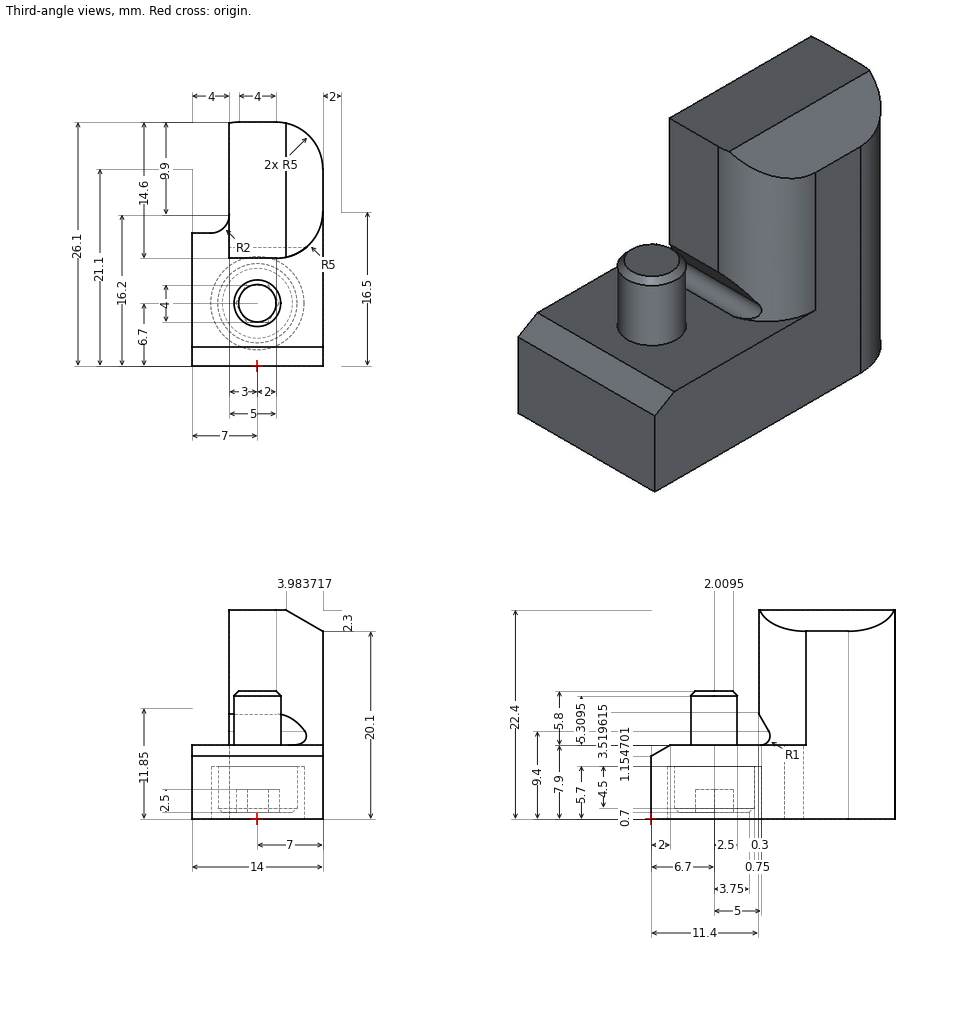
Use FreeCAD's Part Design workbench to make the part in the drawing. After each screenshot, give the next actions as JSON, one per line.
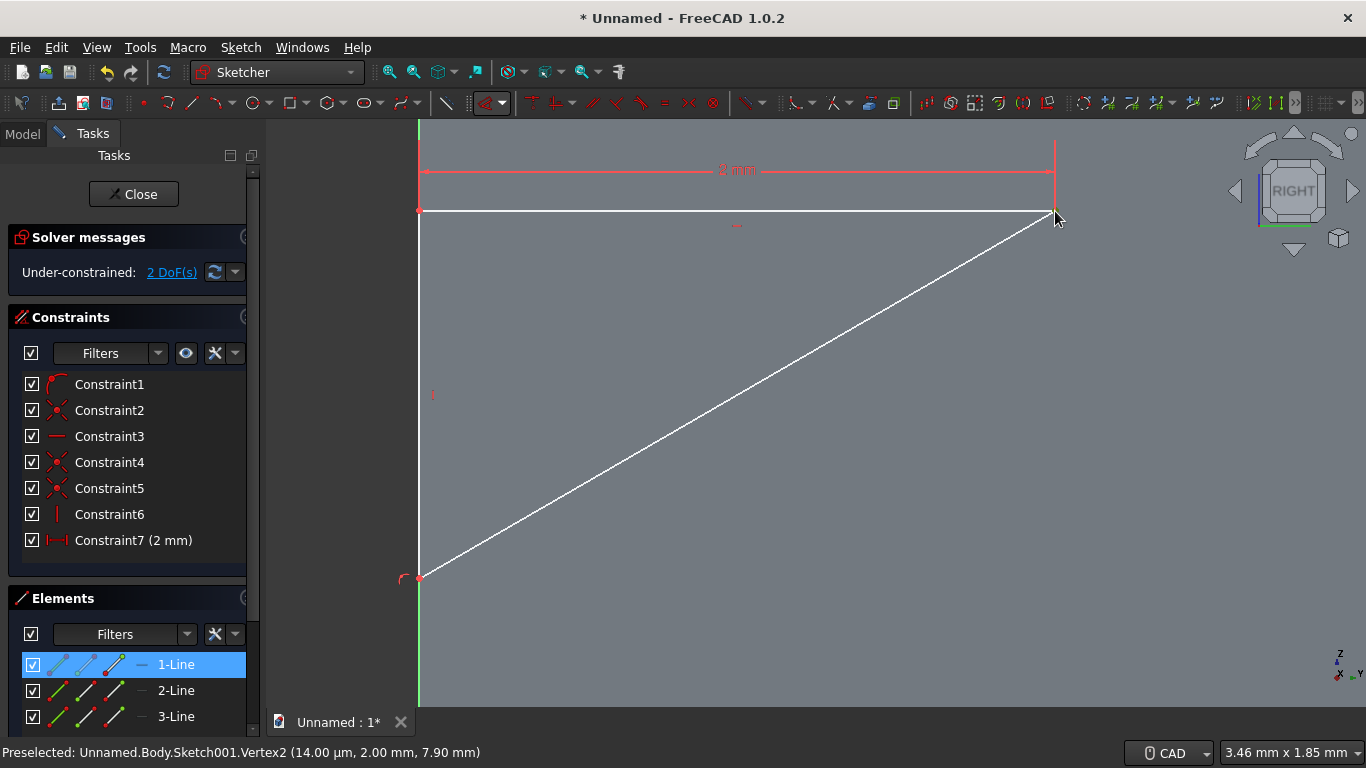
{"action": "left_click", "coordinate": [504, 104]}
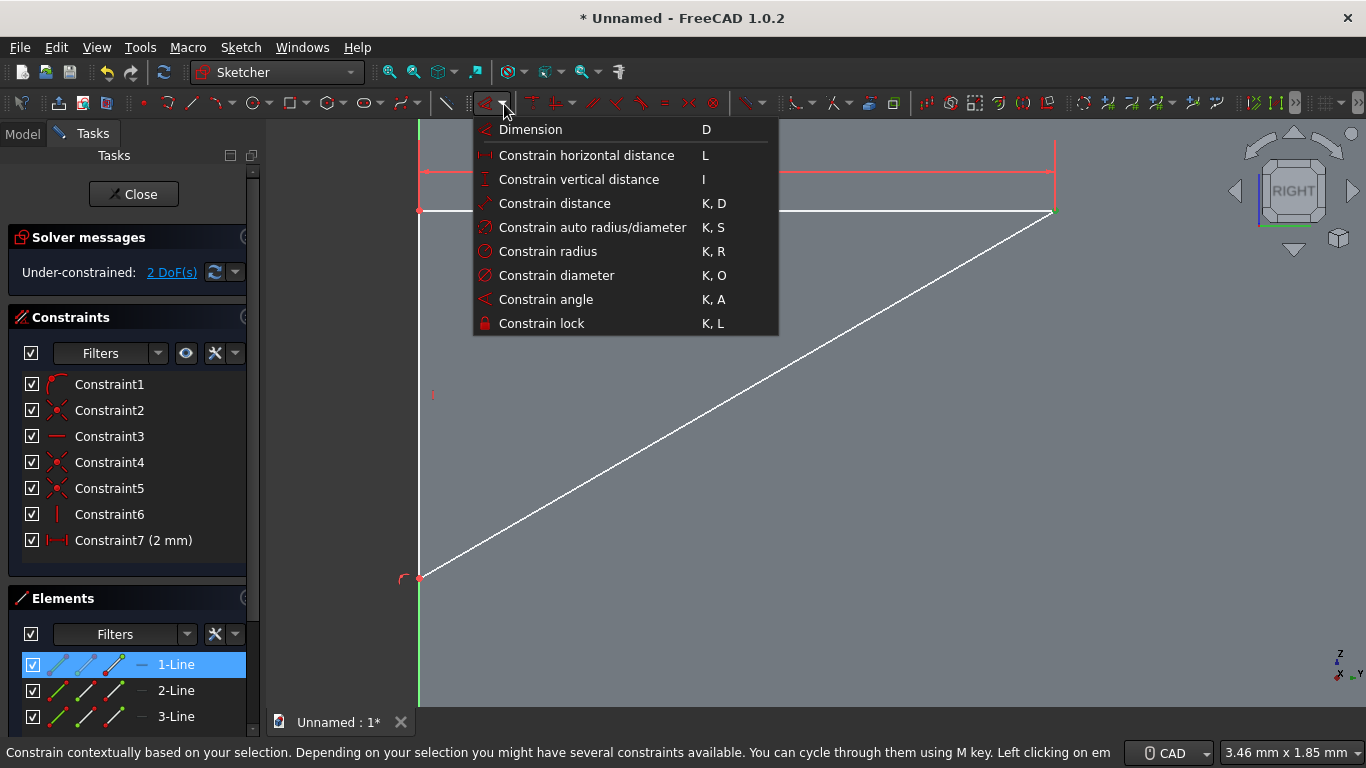
{"action": "left_click", "coordinate": [626, 179]}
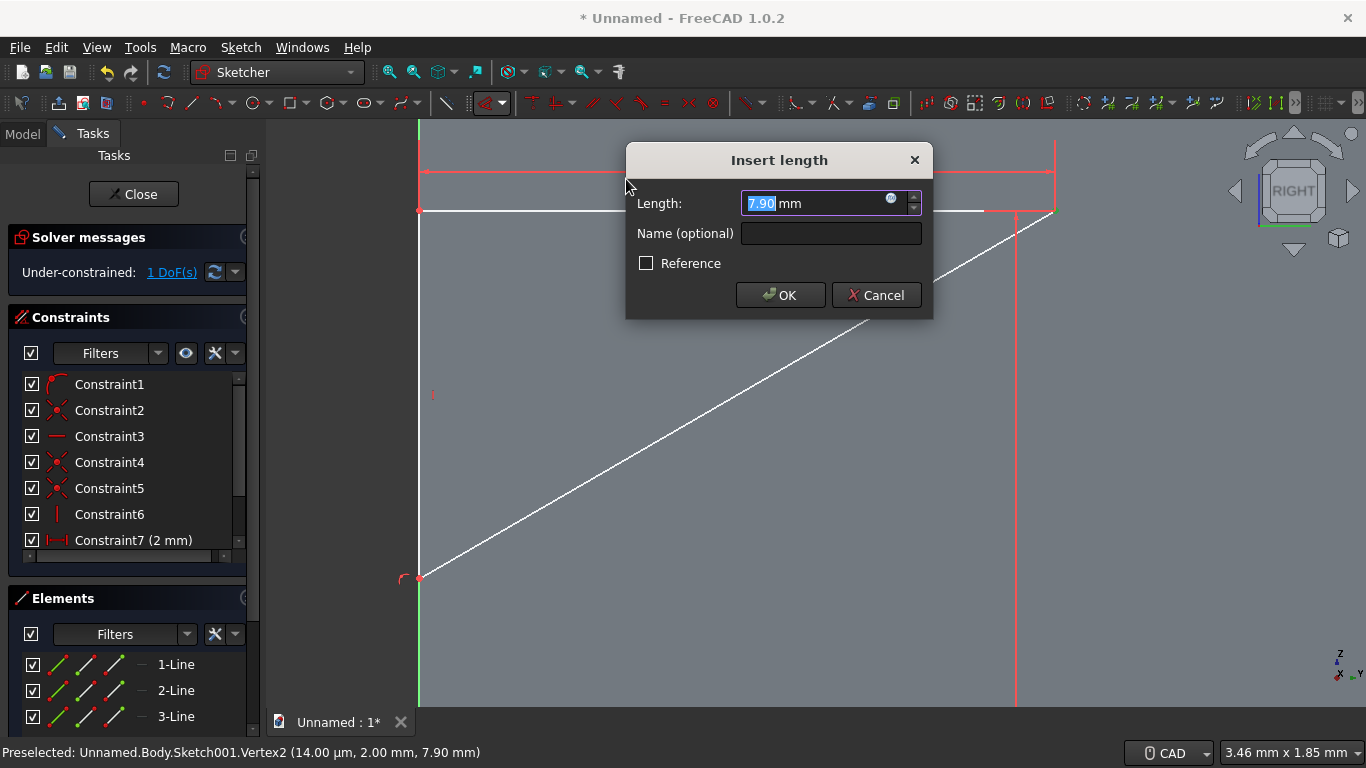
{"action": "type", "text": "7.9"}
{"action": "key", "text": "Return"}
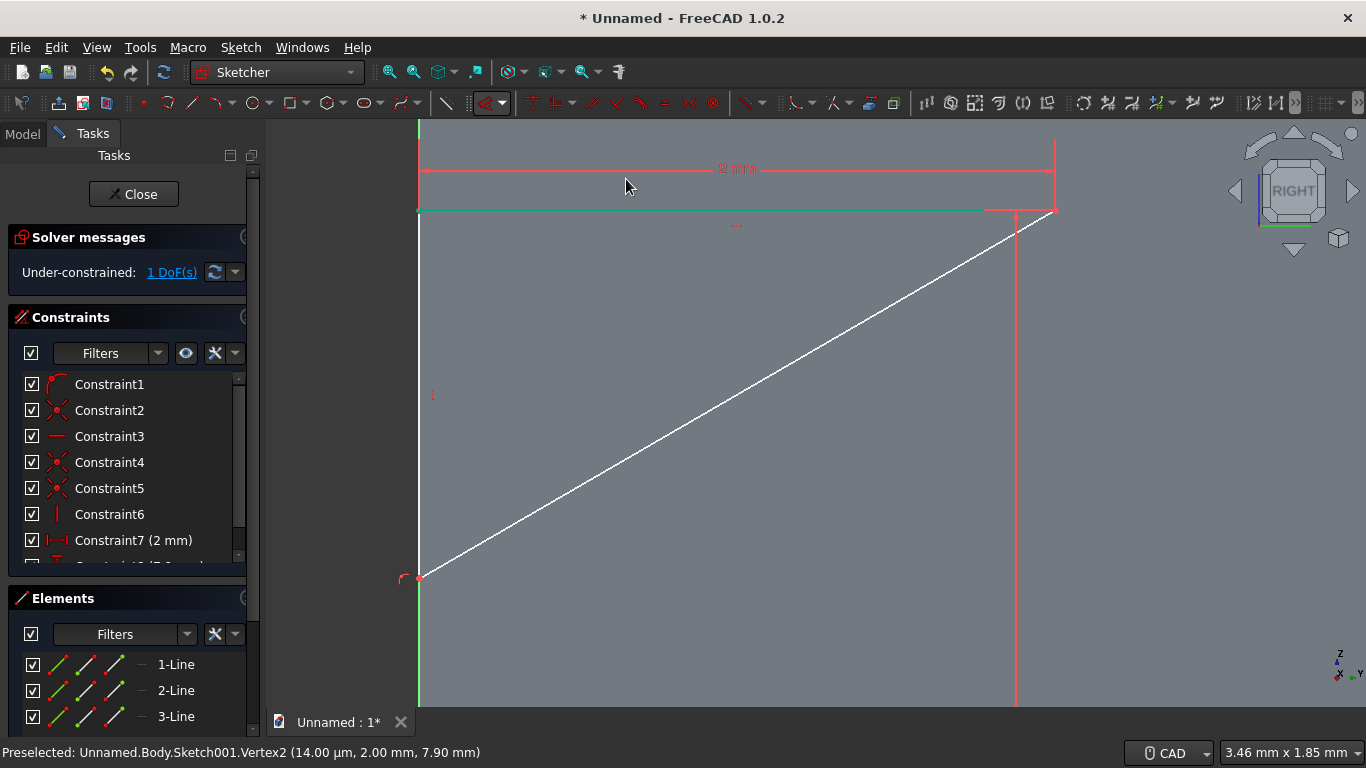
{"action": "left_click", "coordinate": [419, 321]}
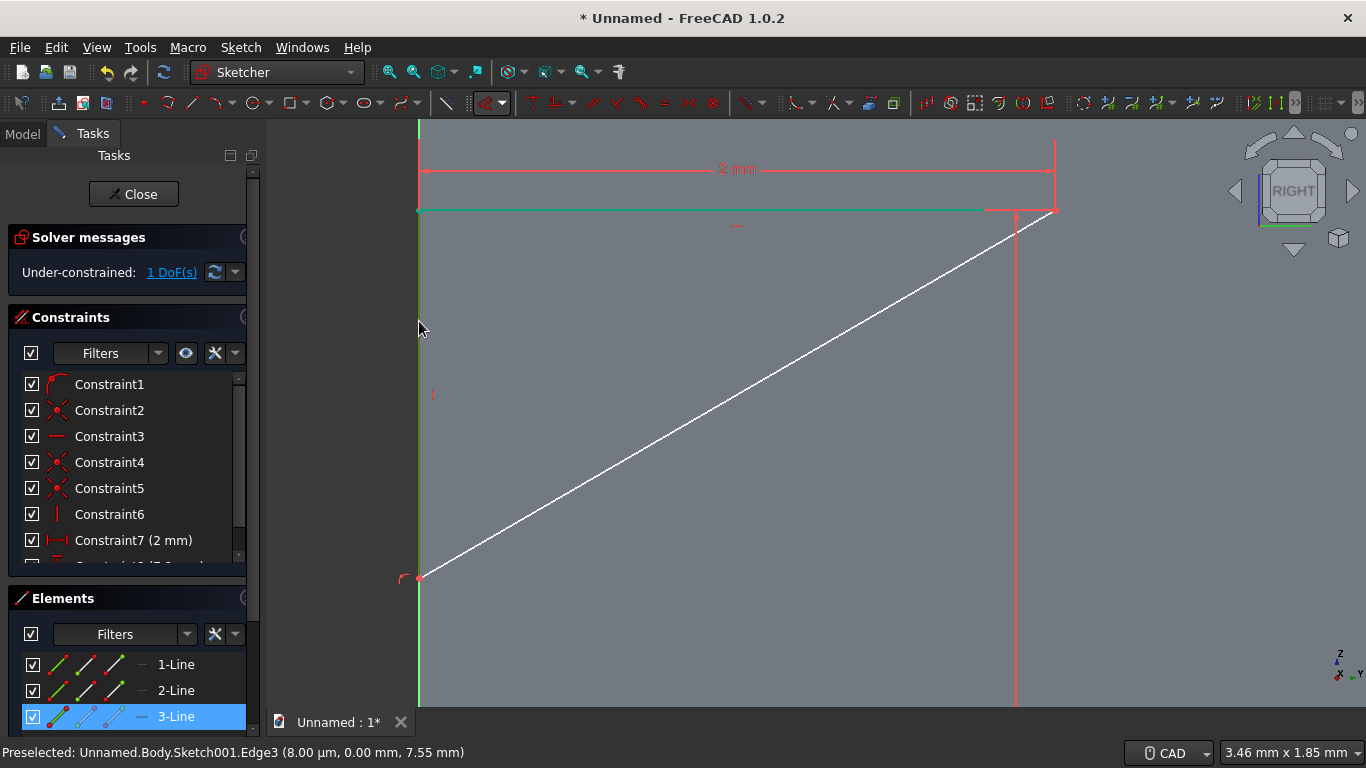
{"action": "left_click", "coordinate": [504, 104]}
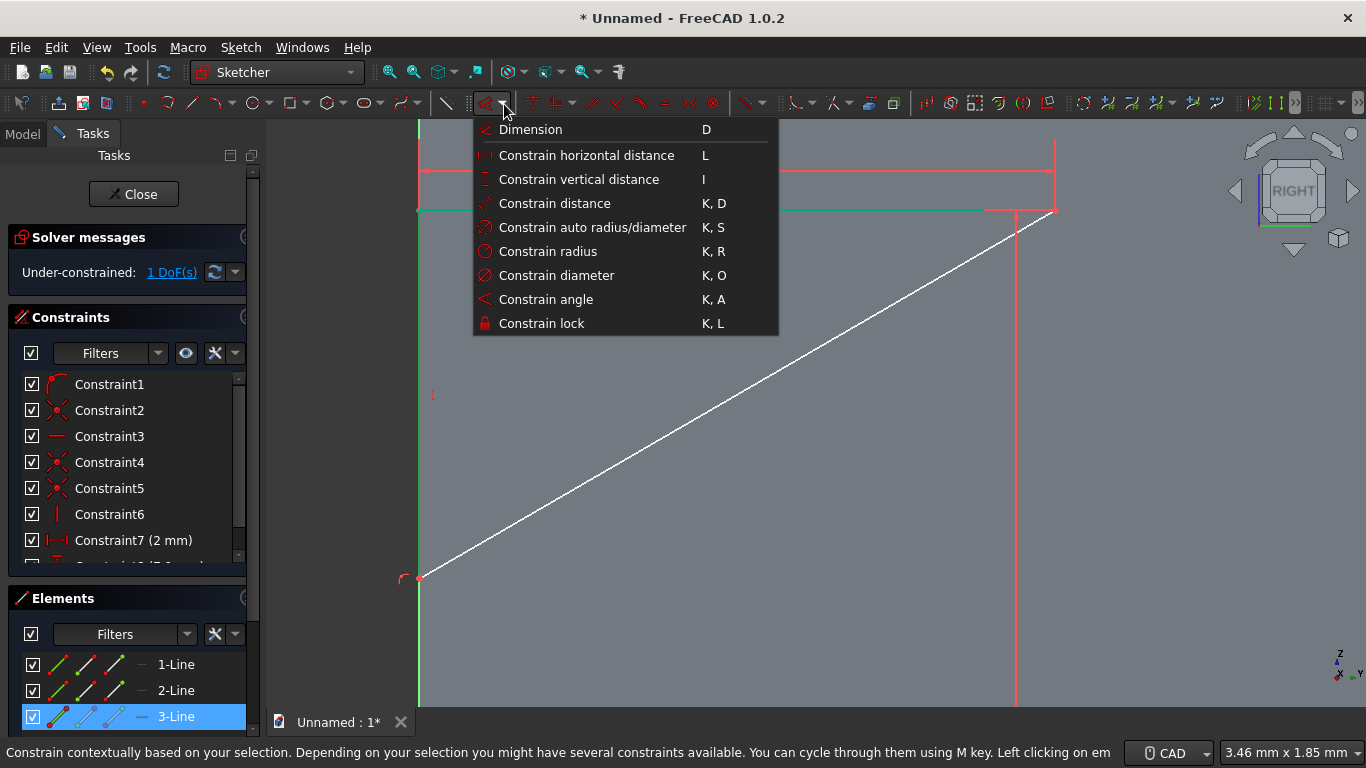
{"action": "left_click", "coordinate": [626, 179]}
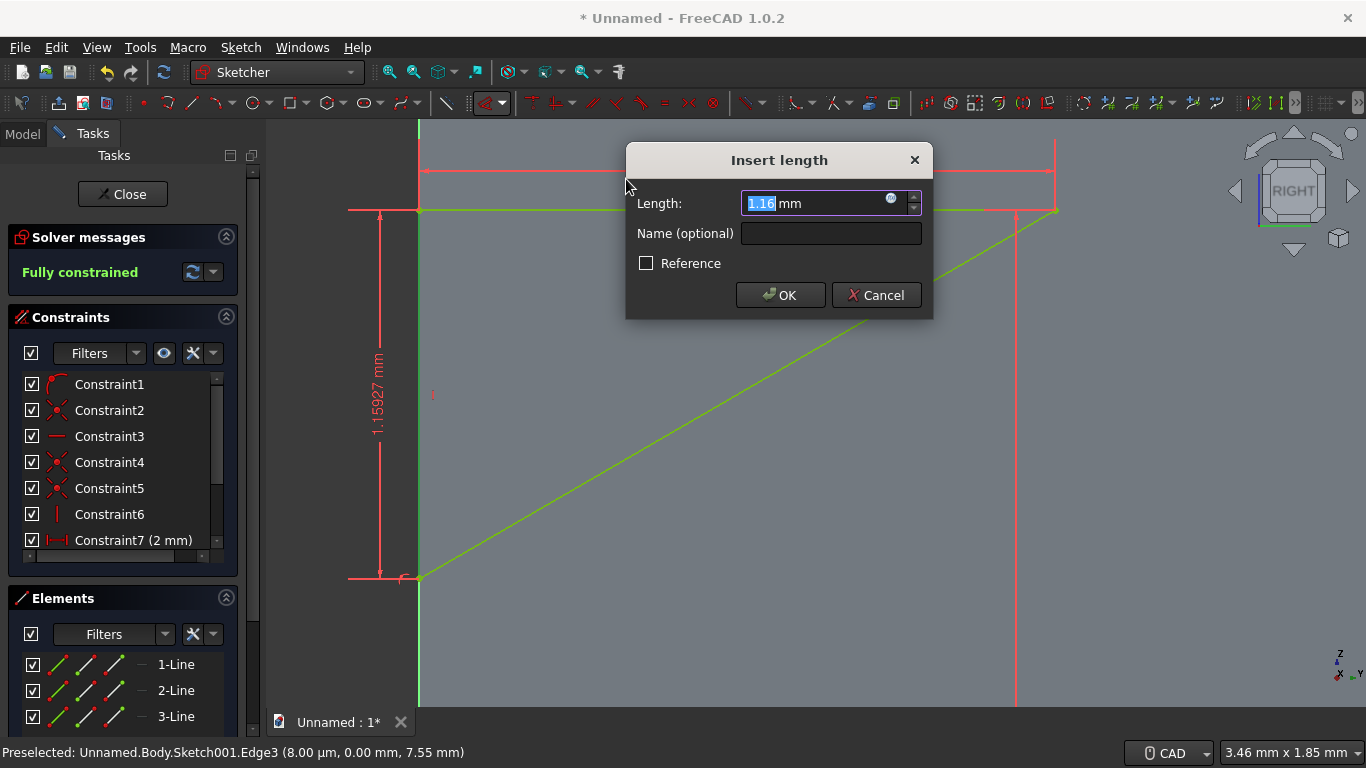
{"action": "type", "text": "1.154701"}
{"action": "key", "text": "Return"}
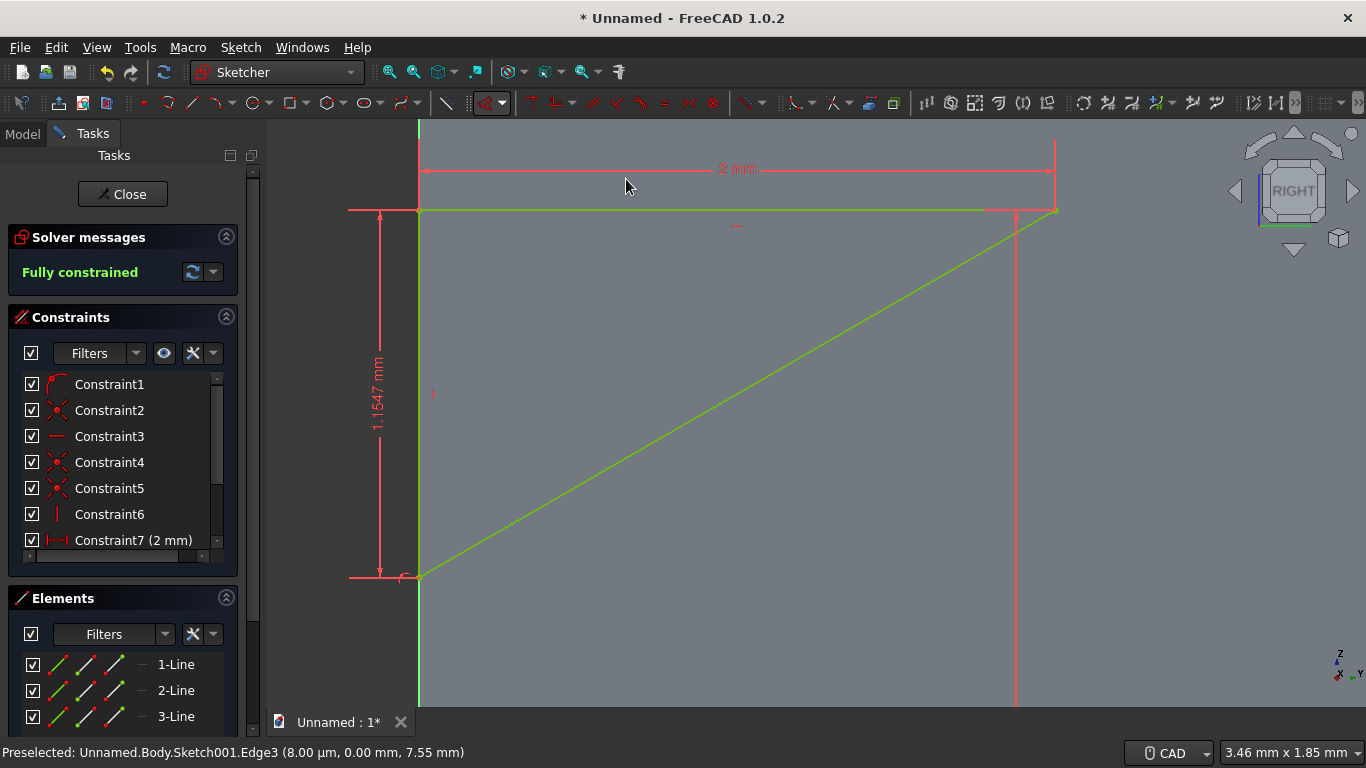
{"action": "left_click", "coordinate": [123, 194]}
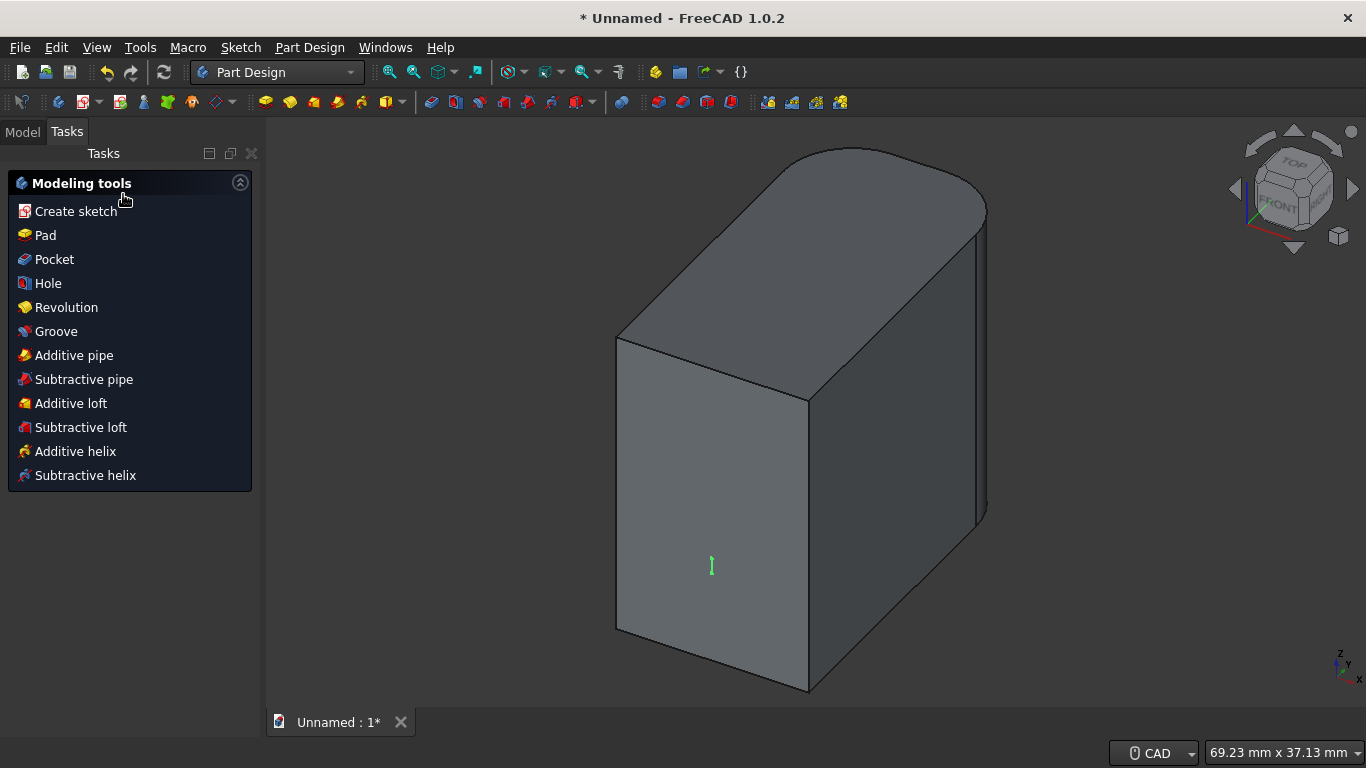
{"action": "left_click", "coordinate": [432, 102]}